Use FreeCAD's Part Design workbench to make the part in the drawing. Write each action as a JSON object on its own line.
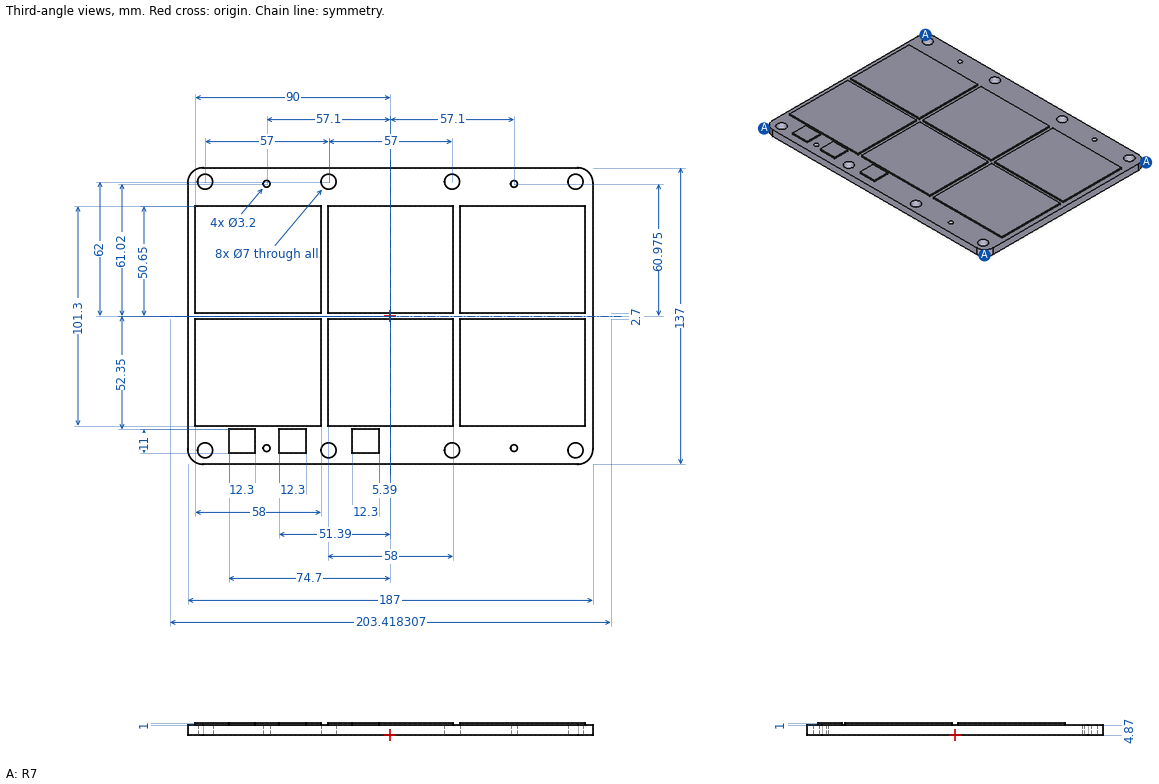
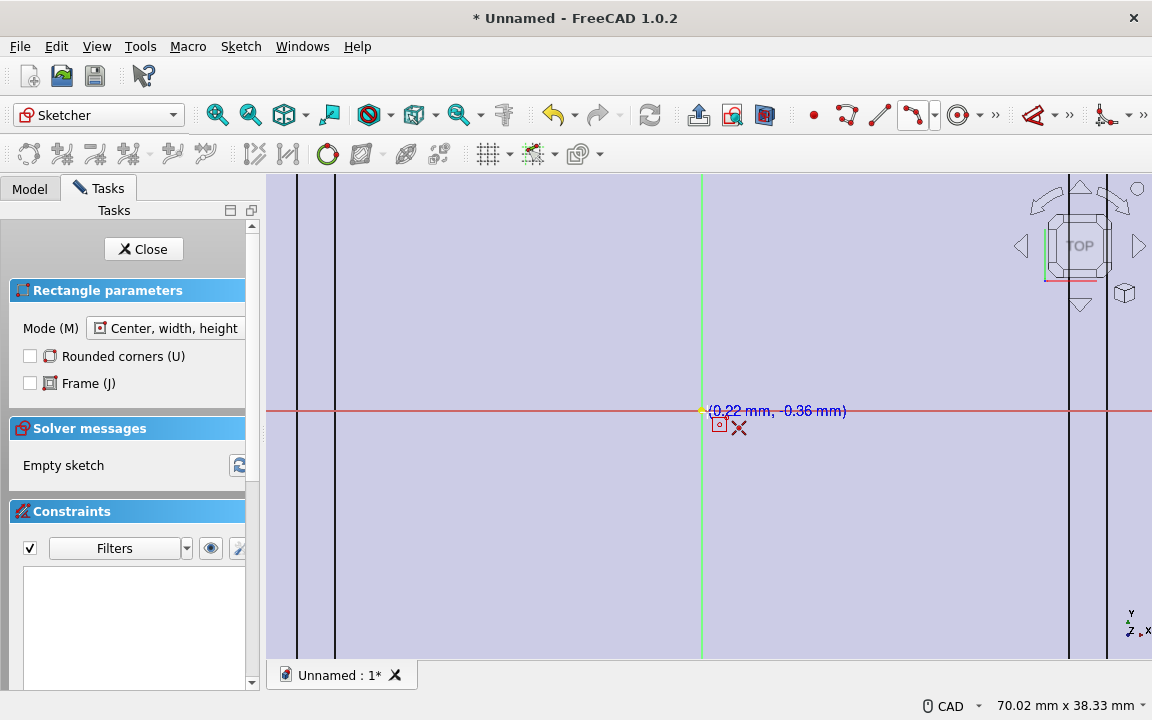
{"action": "scroll", "coordinate": [625, 418], "scroll_direction": "down", "scroll_amount": 8}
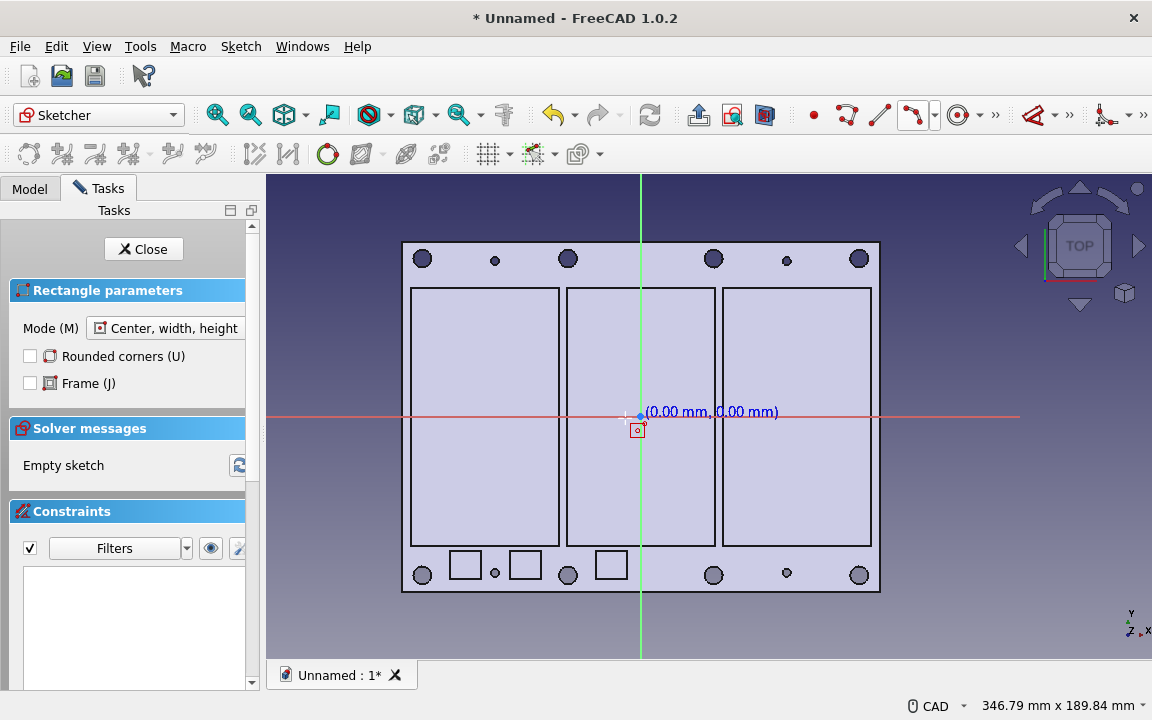
{"action": "left_click", "coordinate": [641, 417]}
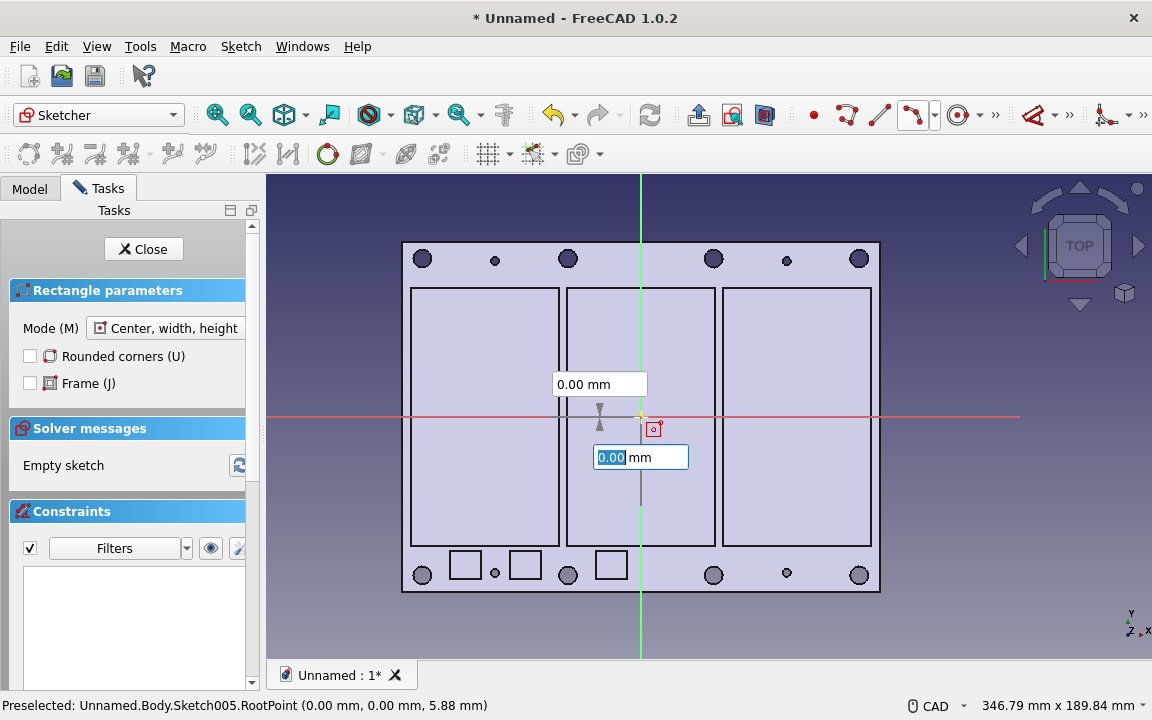
{"action": "scroll", "coordinate": [901, 414], "scroll_direction": "up", "scroll_amount": 8}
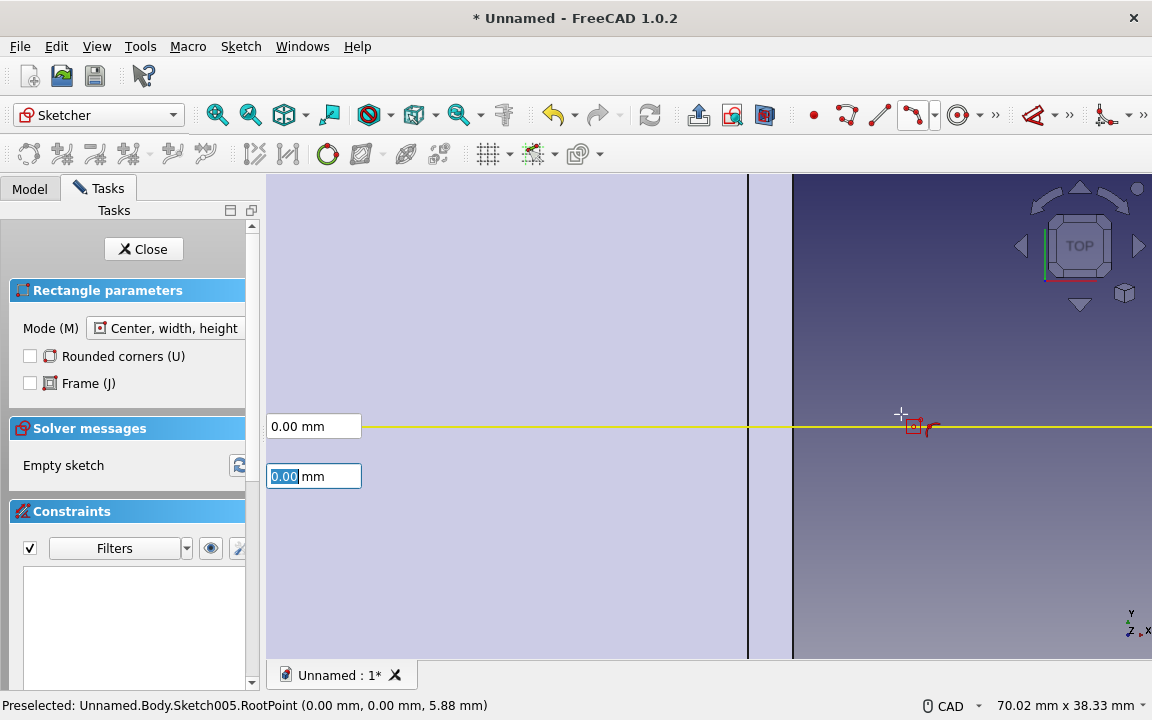
{"action": "left_click", "coordinate": [896, 410]}
{"action": "key", "text": "Escape"}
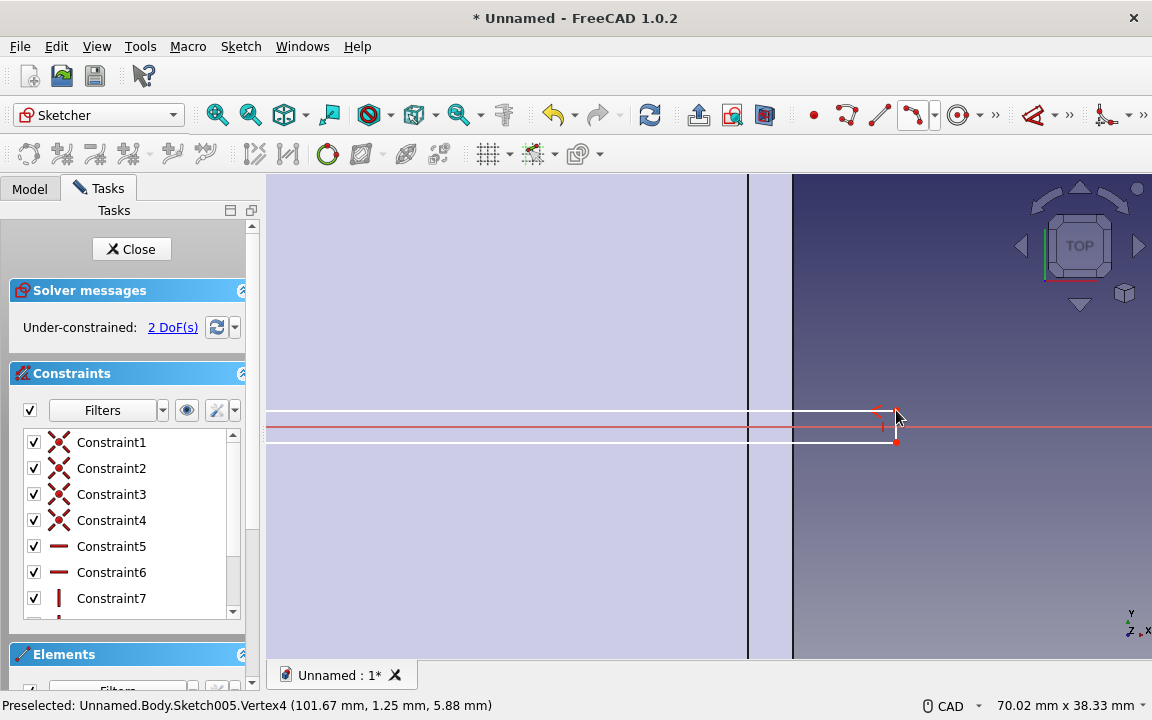
{"action": "key", "text": "d"}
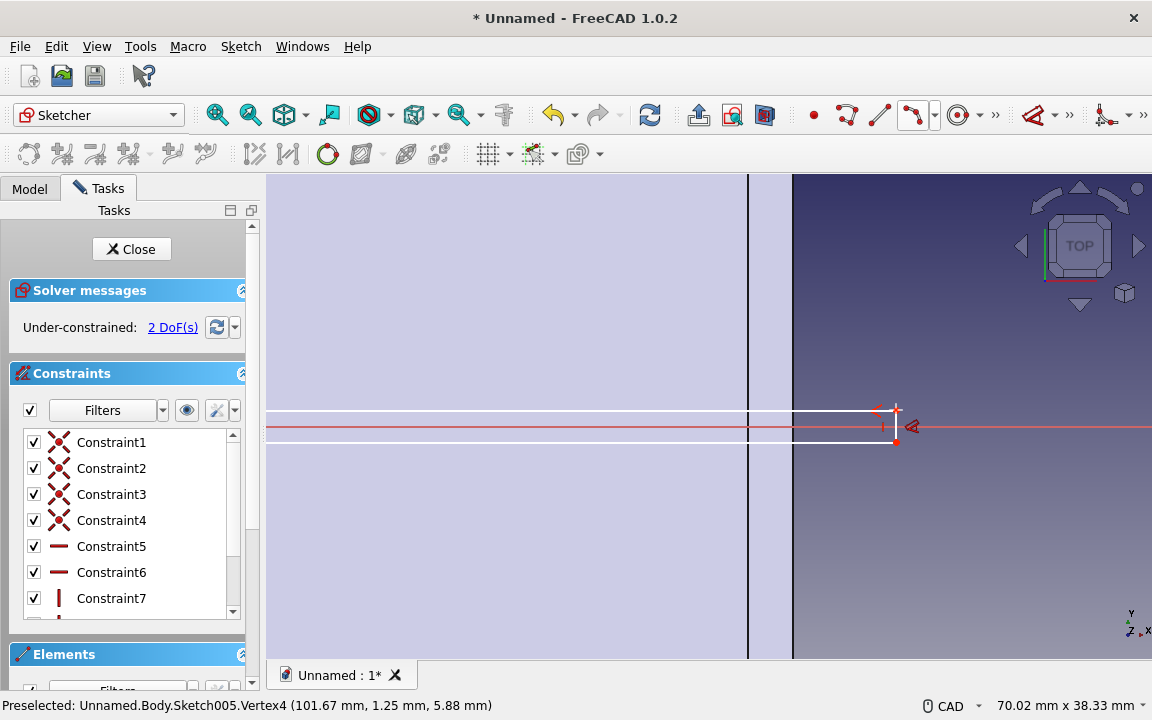
{"action": "left_click", "coordinate": [896, 430]}
{"action": "left_click", "coordinate": [930, 420]}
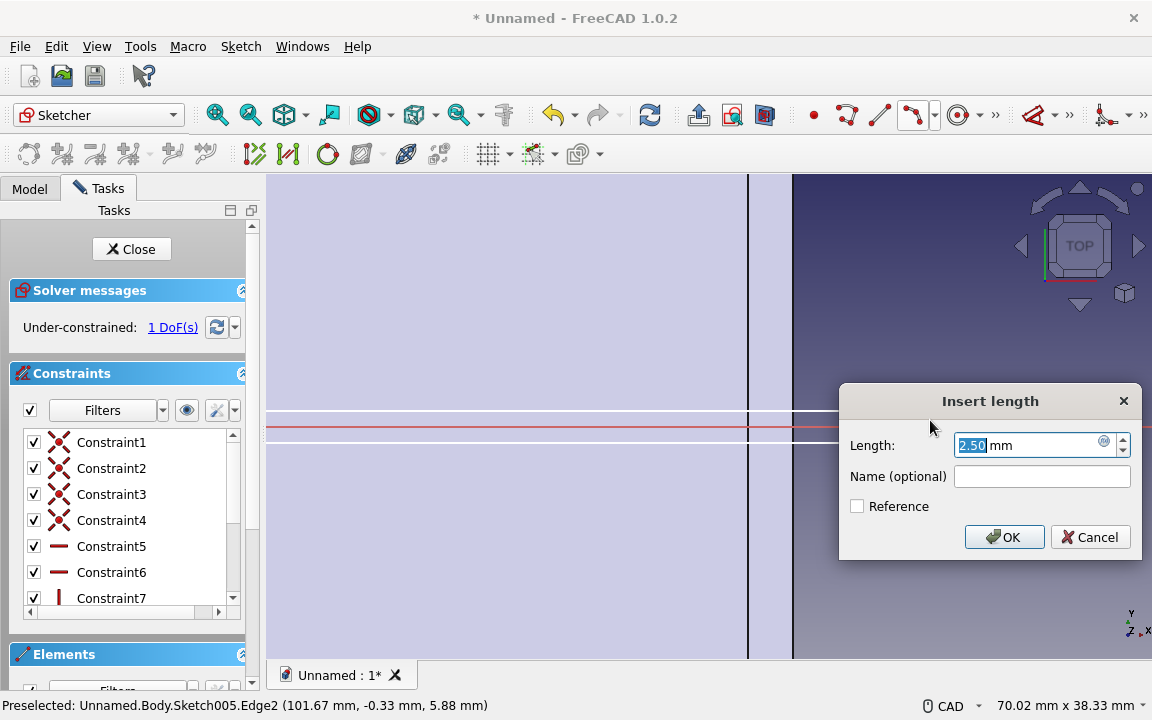
{"action": "type", "text": "2.7"}
{"action": "key", "text": "Return"}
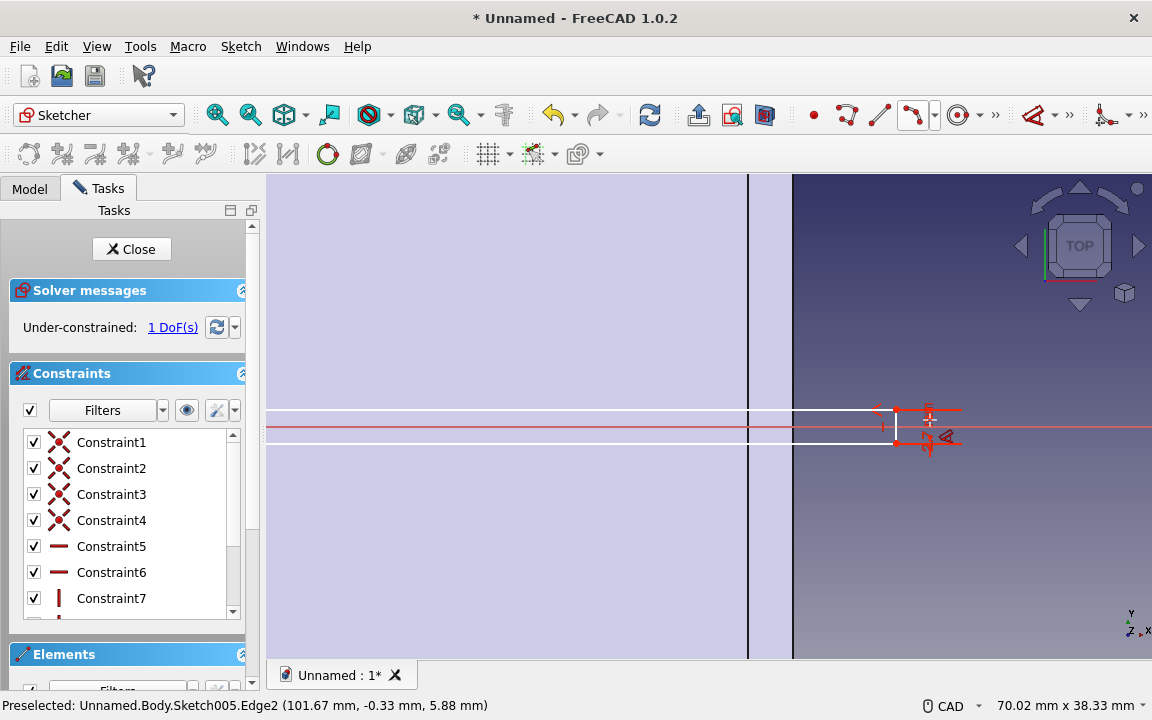
{"action": "left_click", "coordinate": [381, 444]}
{"action": "left_click", "coordinate": [595, 478]}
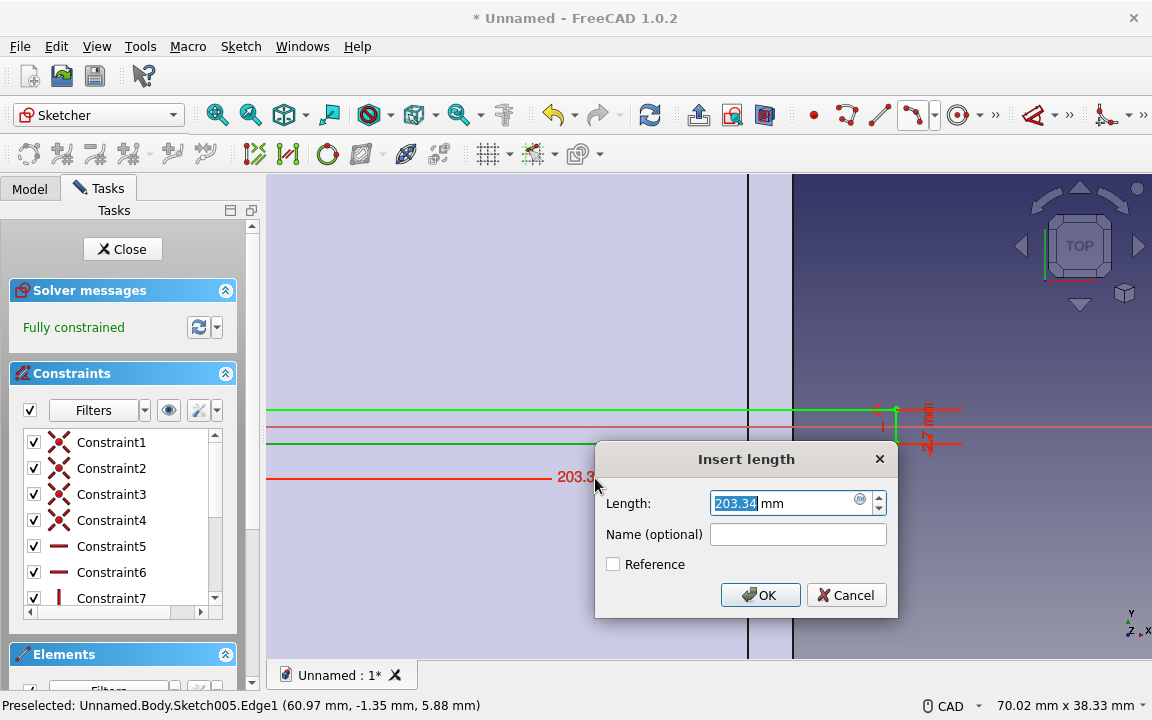
{"action": "type", "text": "203.418307"}
{"action": "key", "text": "Return"}
{"action": "key", "text": "Escape"}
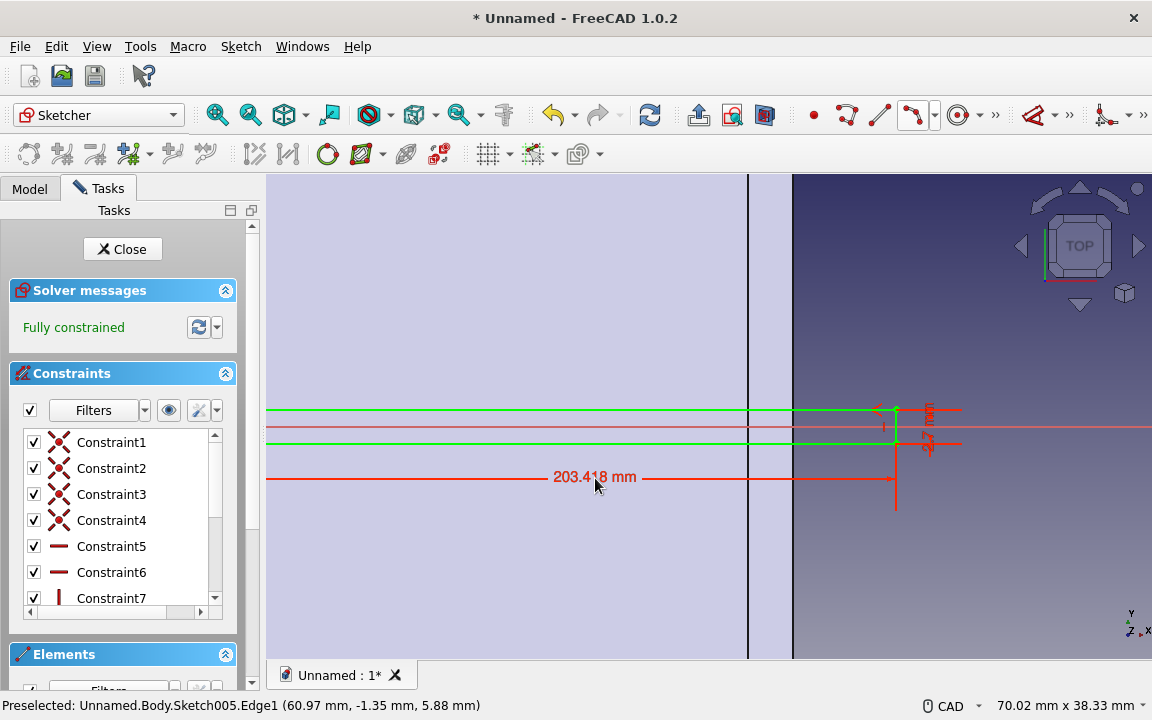
{"action": "left_click", "coordinate": [123, 249]}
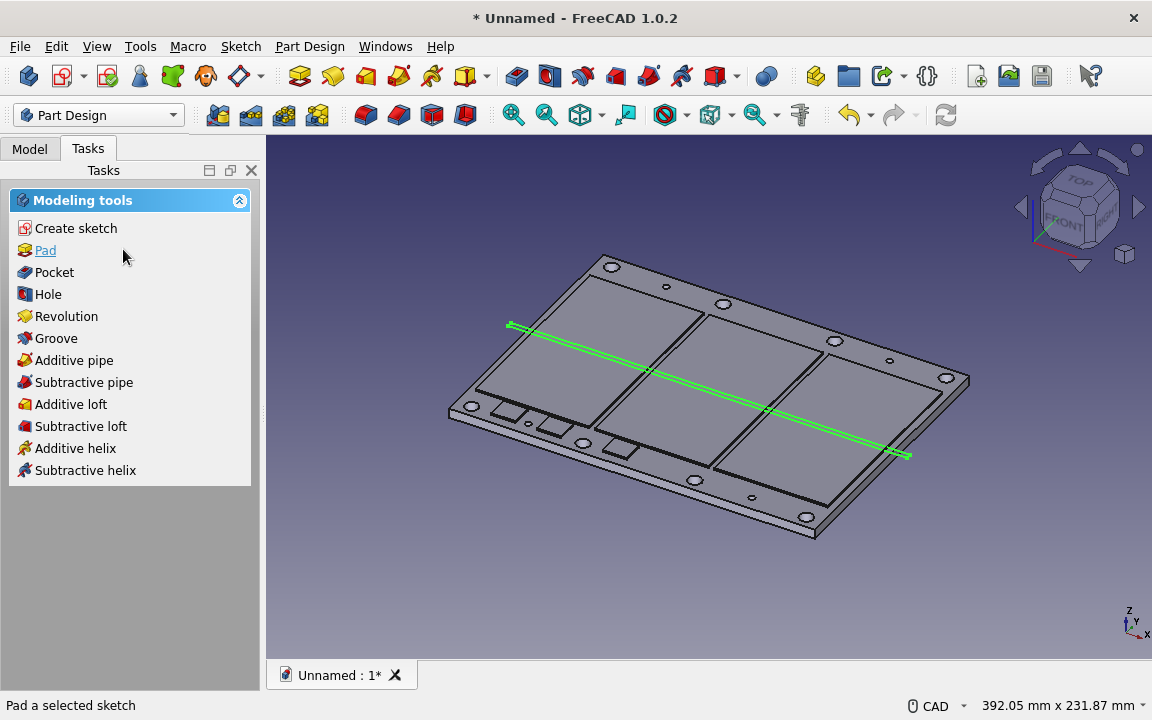
{"action": "left_click", "coordinate": [517, 76]}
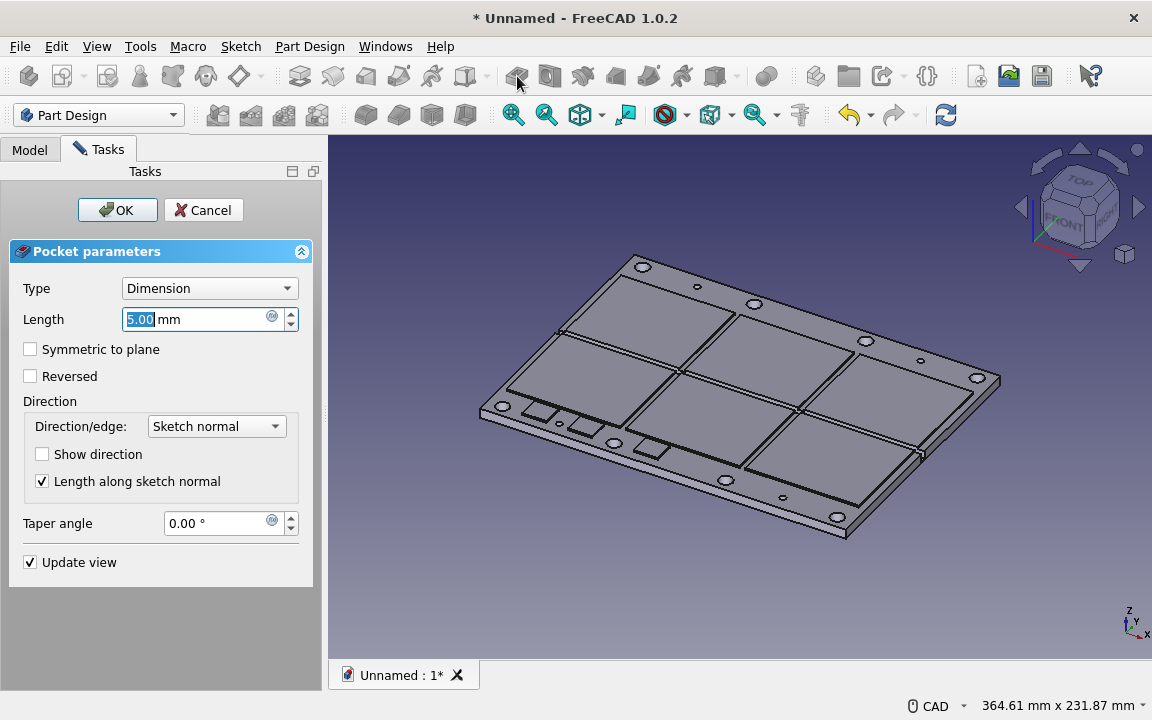
{"action": "type", "text": "1"}
{"action": "key", "text": "Tab"}